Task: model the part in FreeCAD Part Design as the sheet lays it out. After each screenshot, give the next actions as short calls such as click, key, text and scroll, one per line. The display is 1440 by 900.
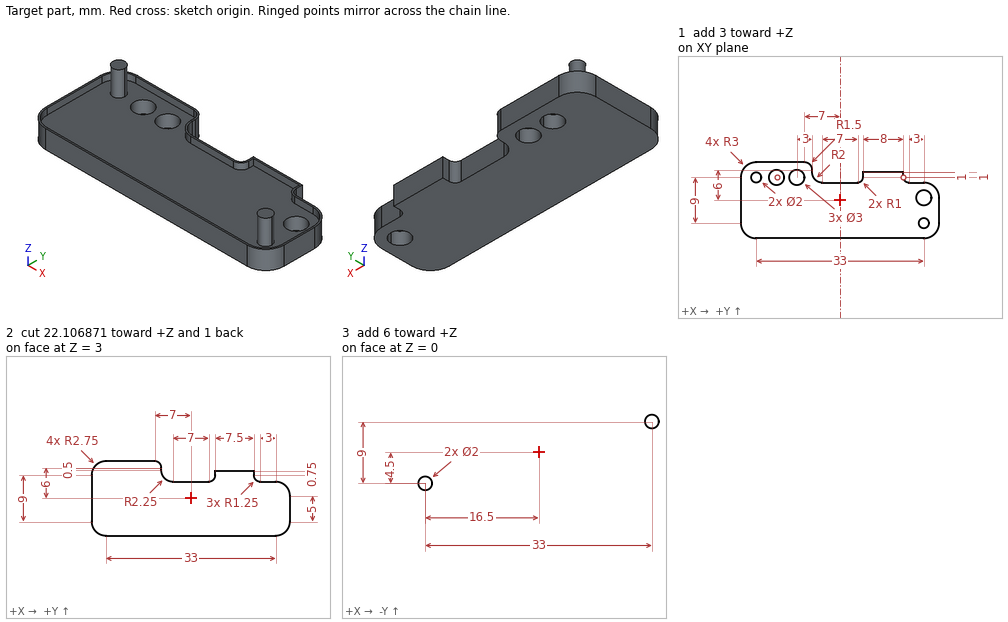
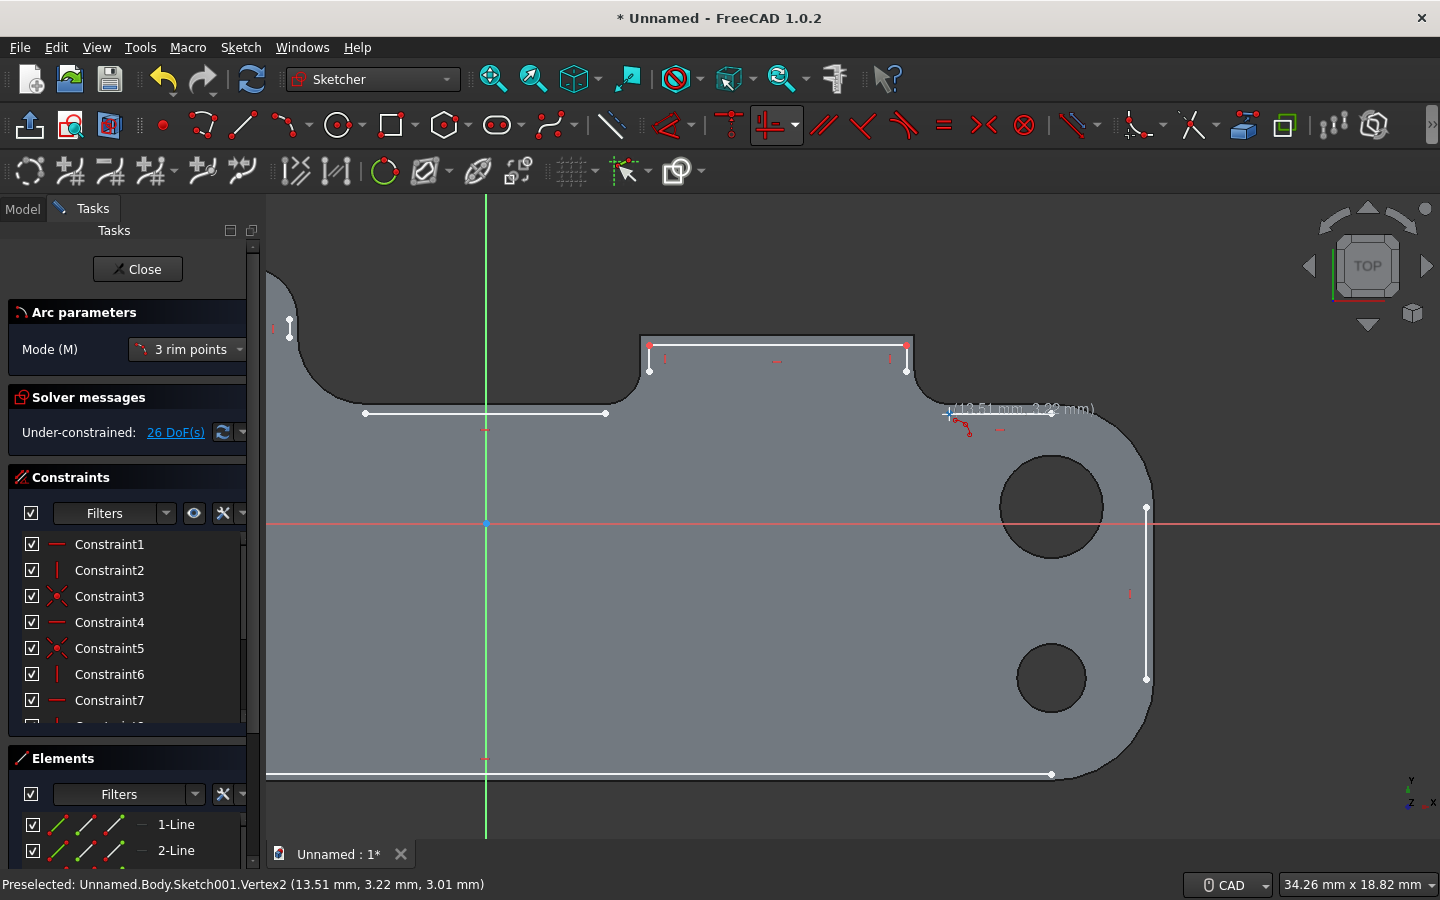
scroll(906, 370, up, 2)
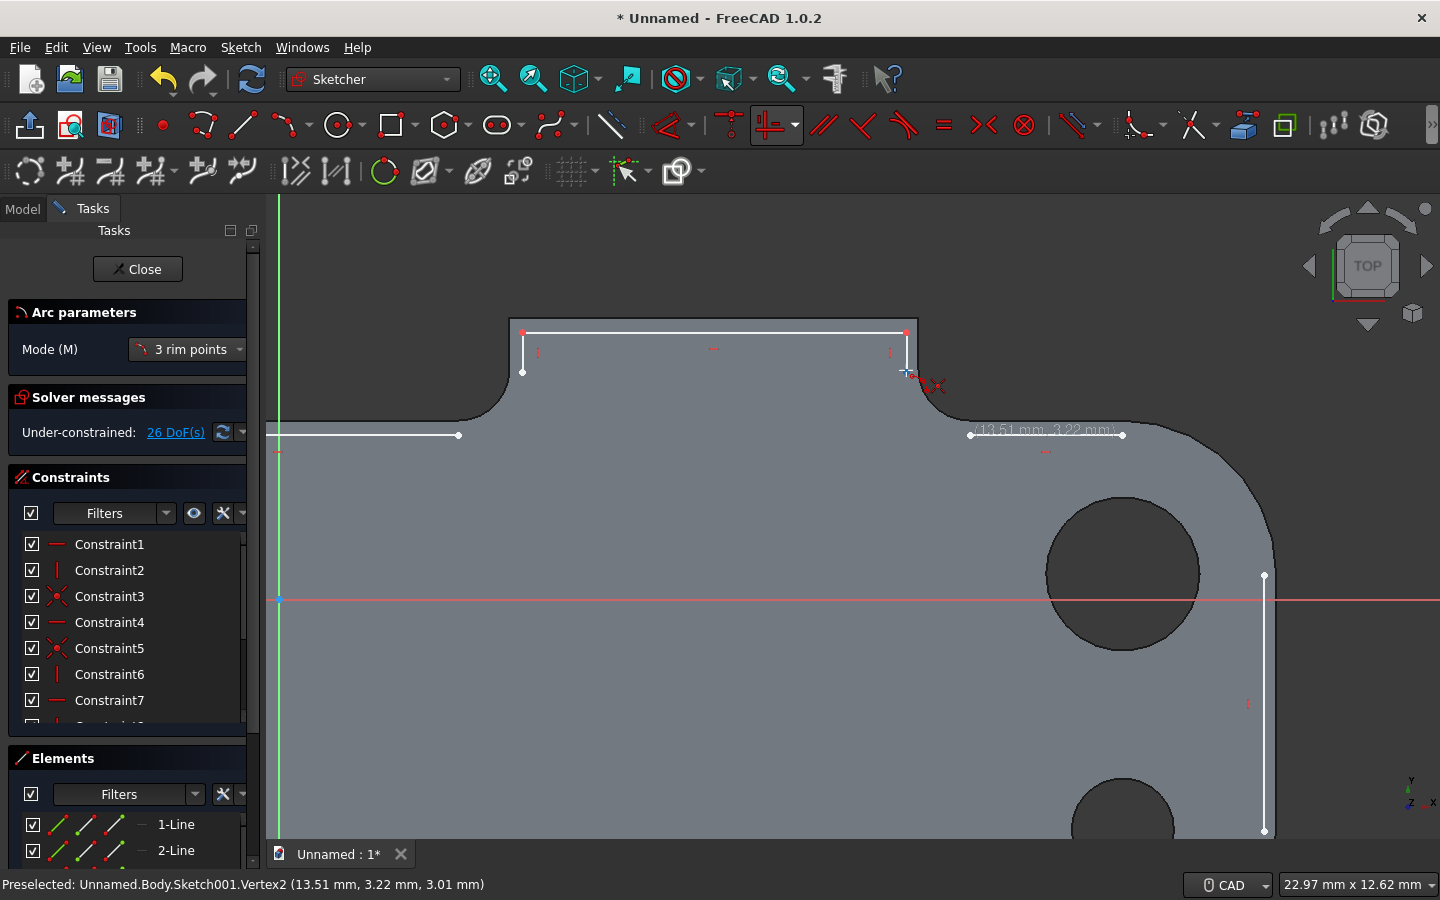
click(907, 372)
click(924, 415)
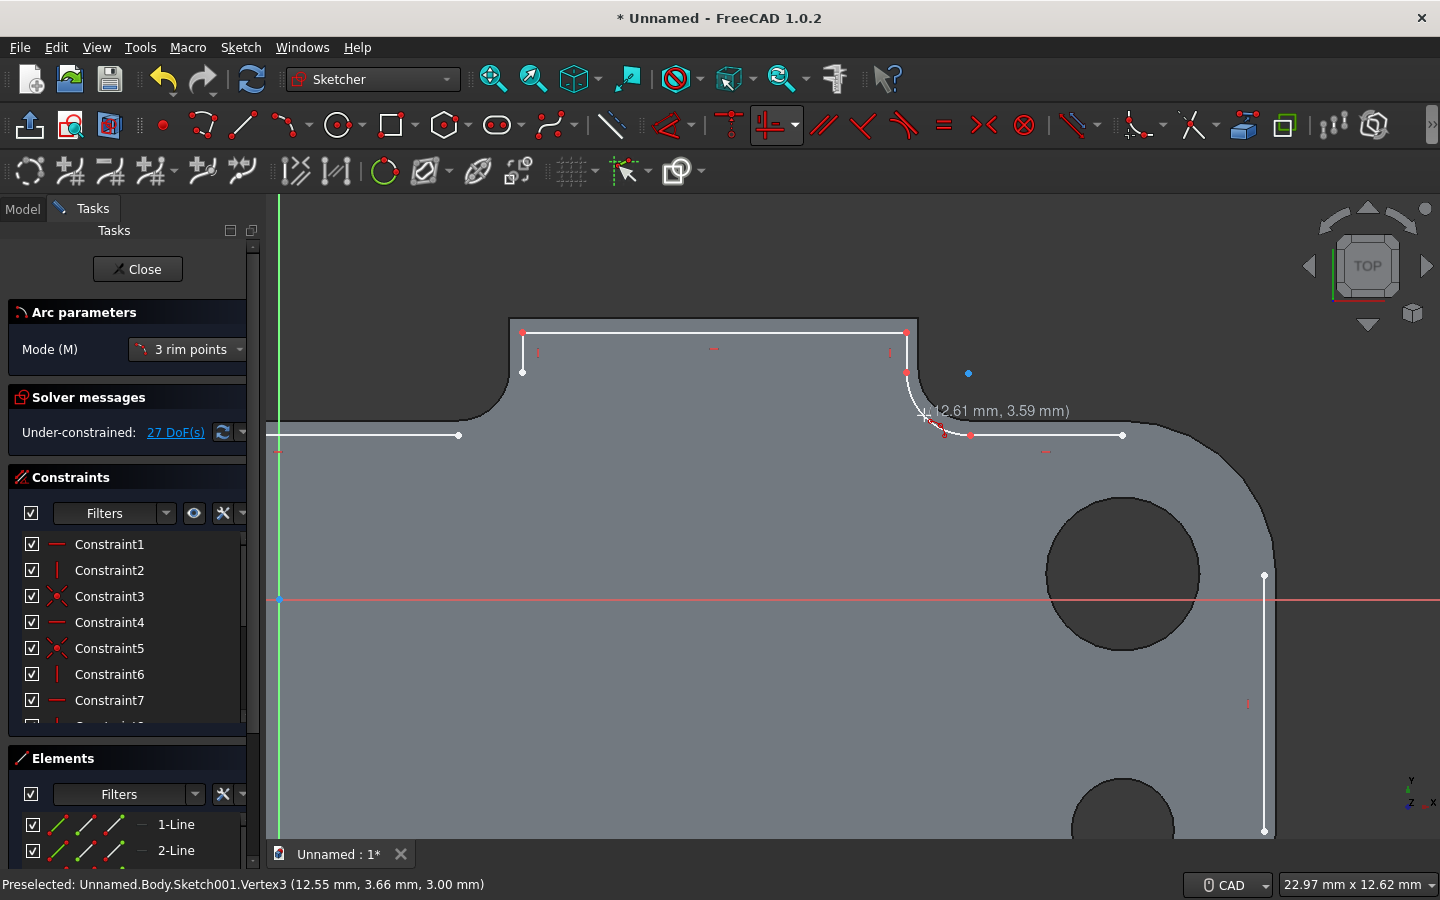
click(523, 373)
click(458, 435)
click(504, 415)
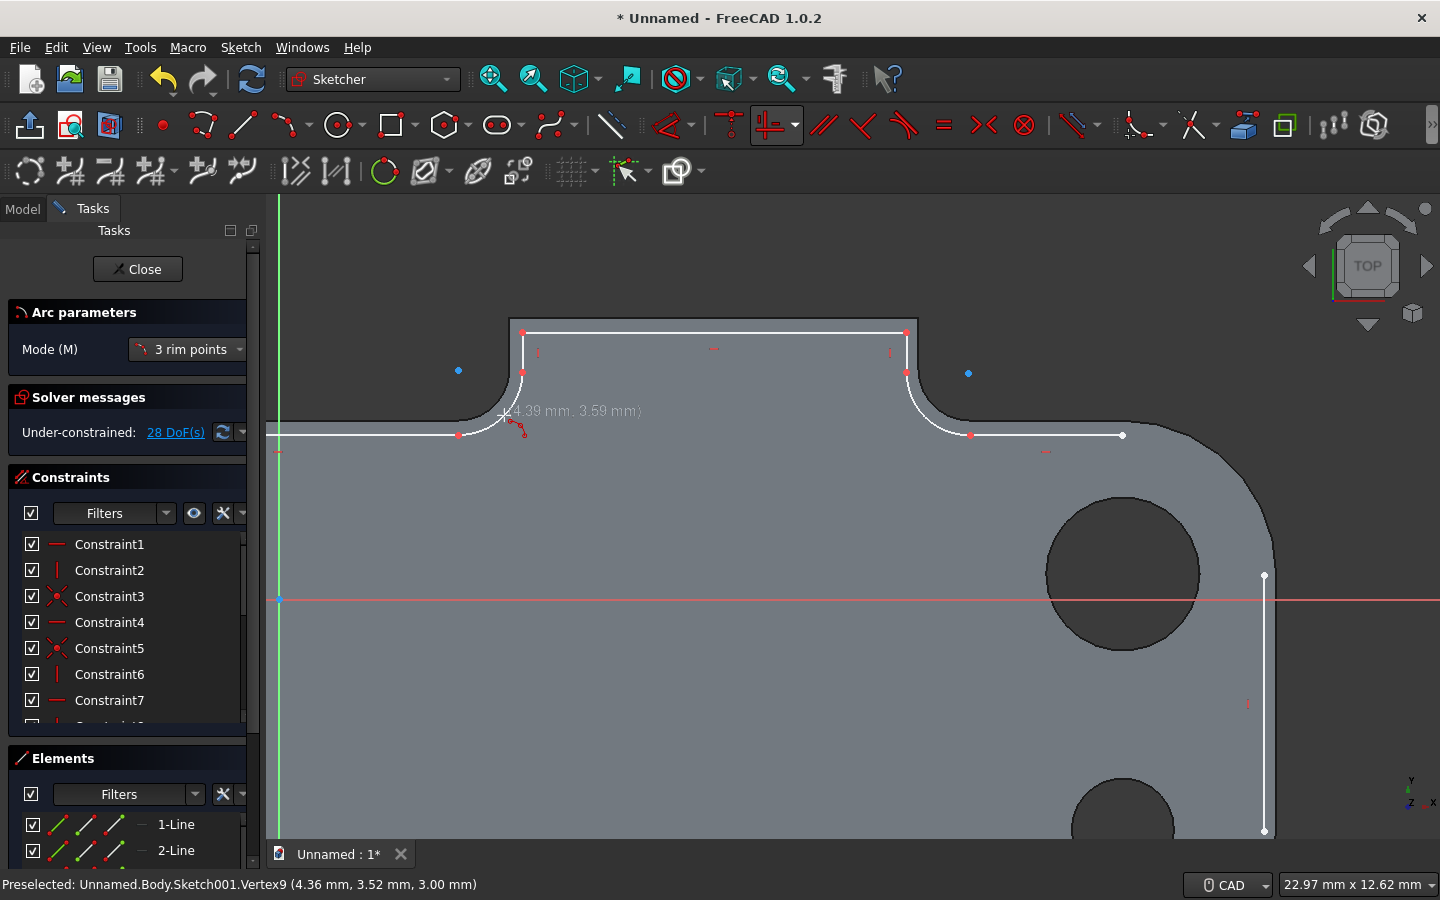
scroll(1078, 468, down, 5)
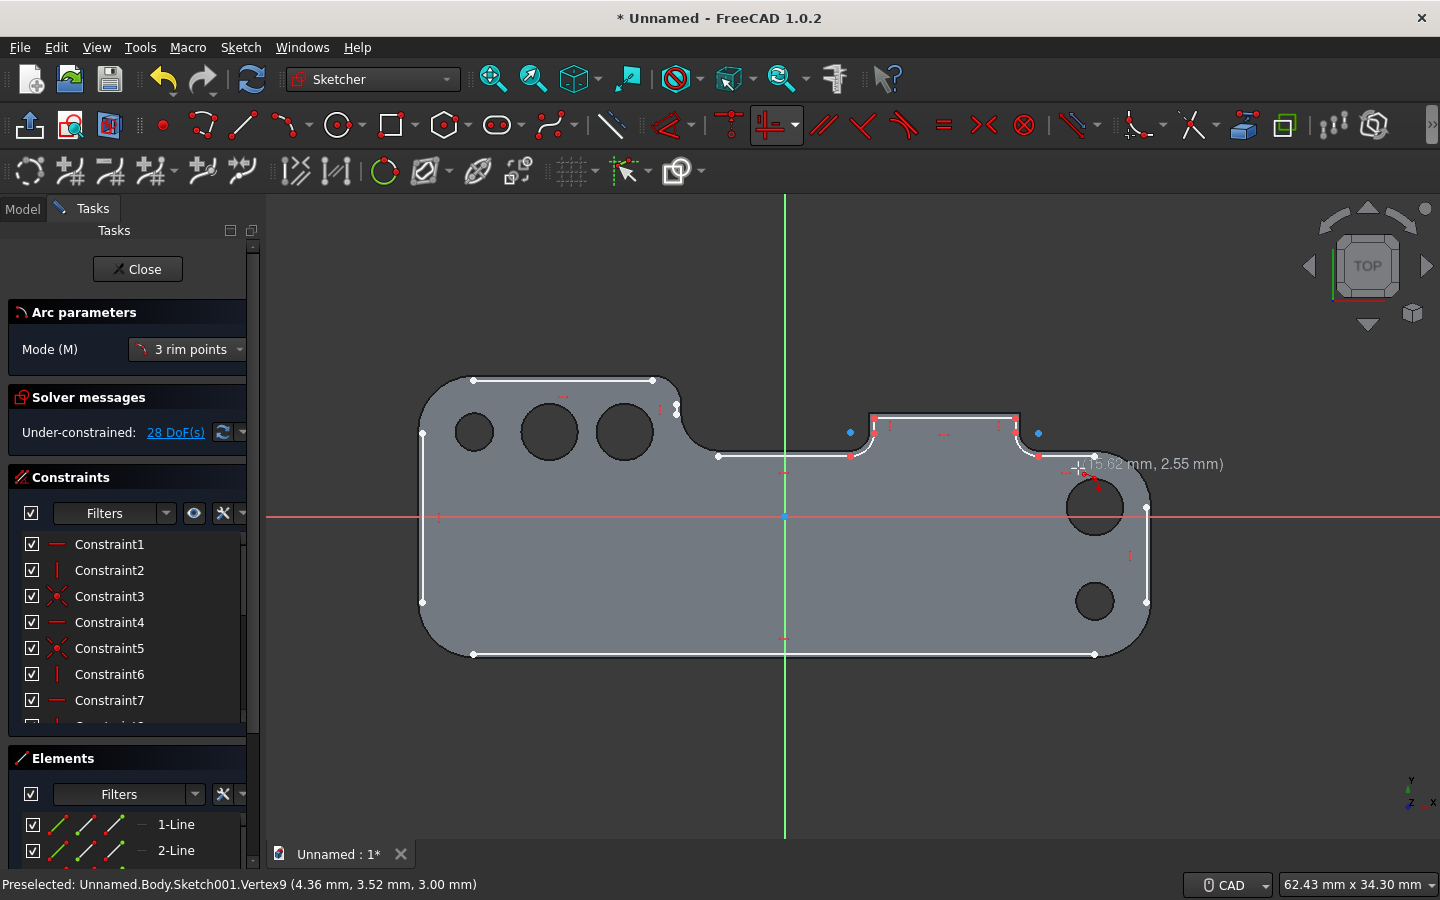
click(719, 456)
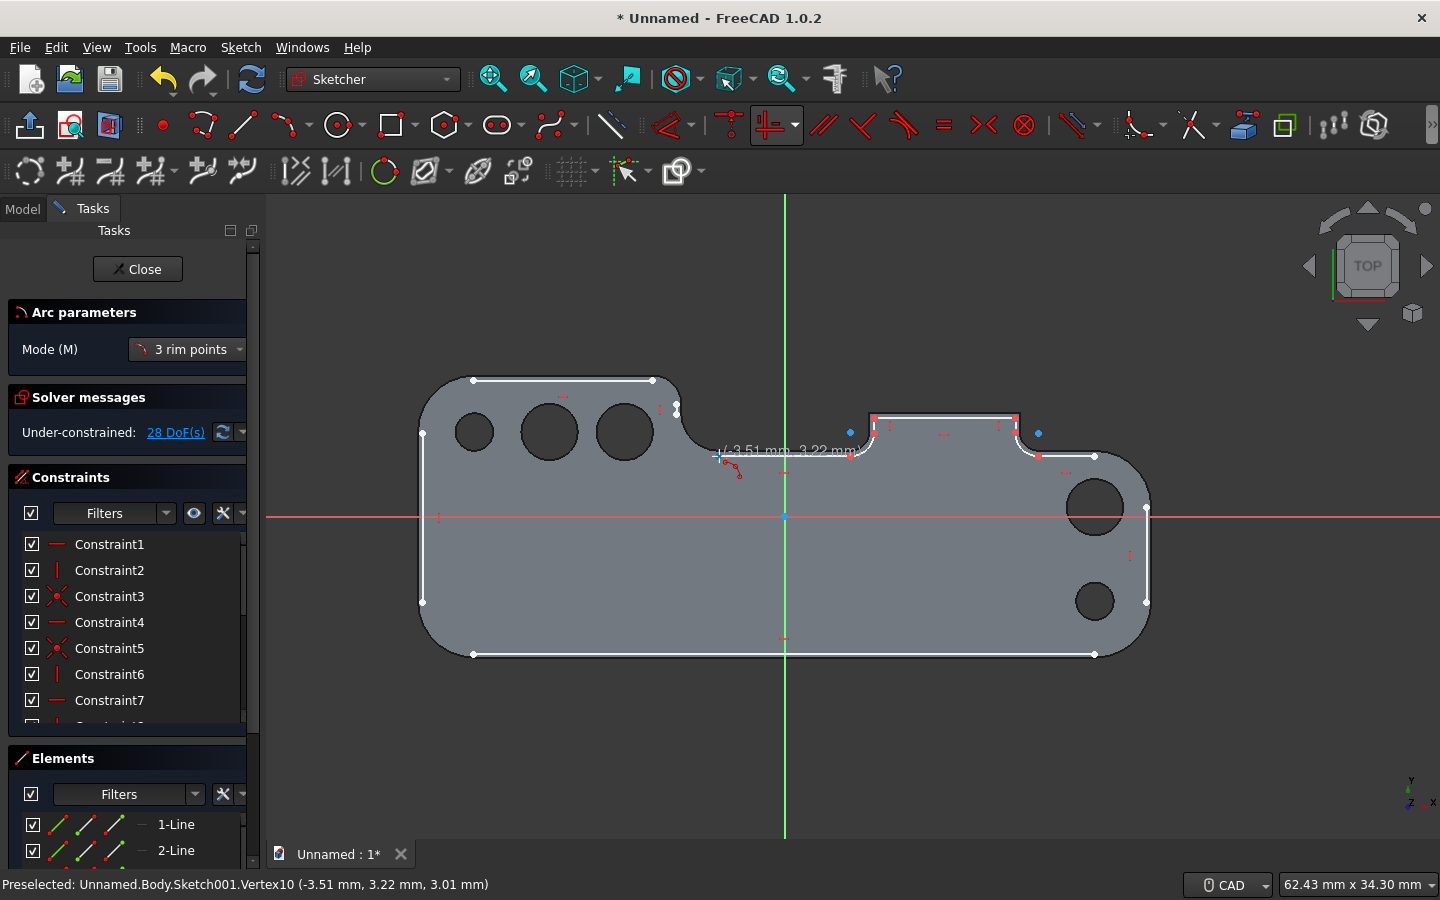
scroll(677, 413, up, 7)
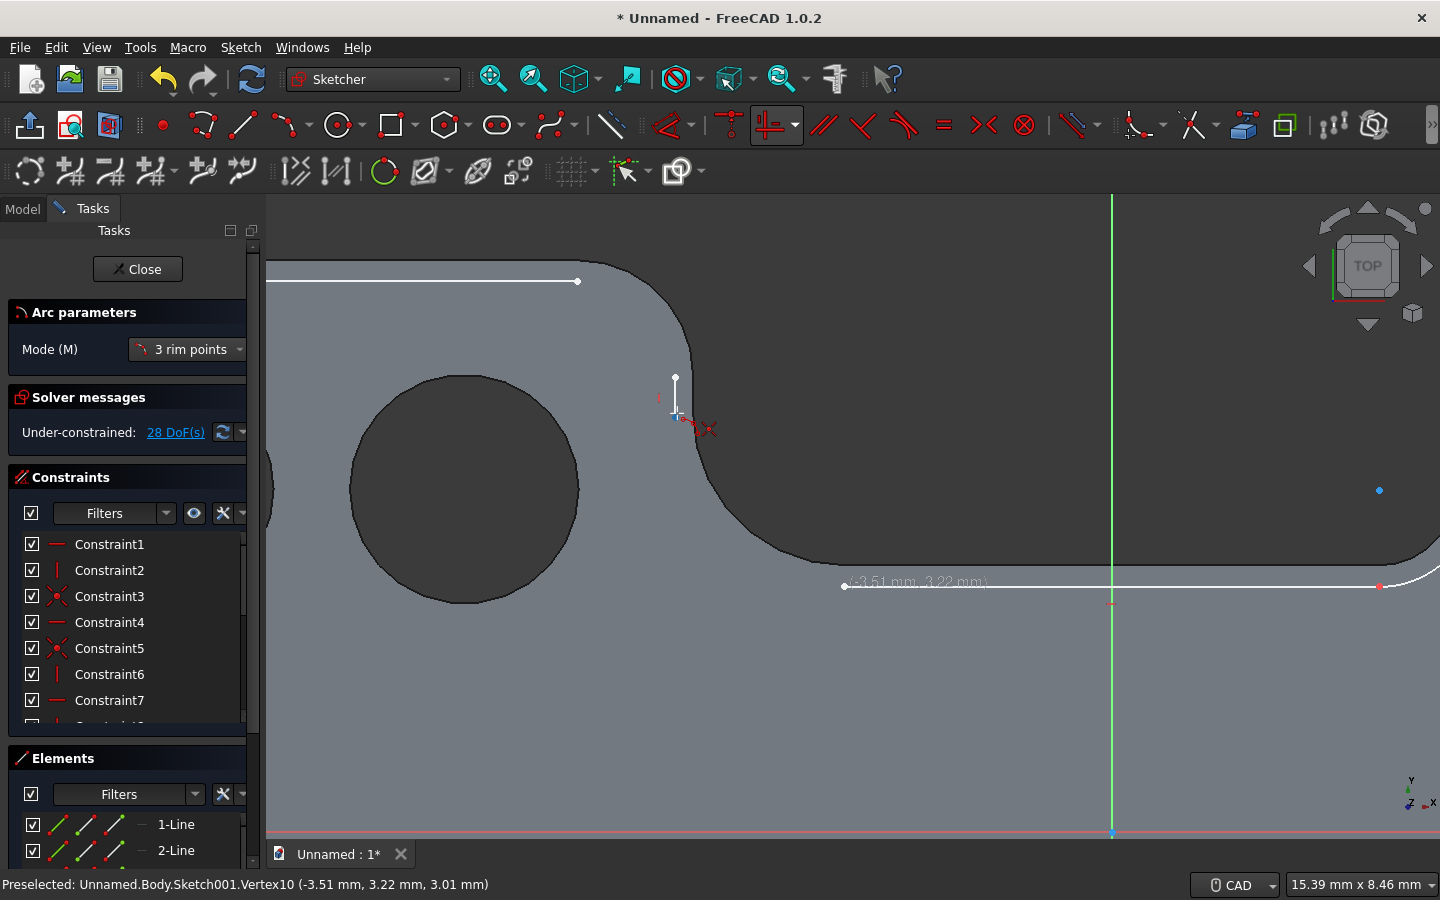
click(675, 418)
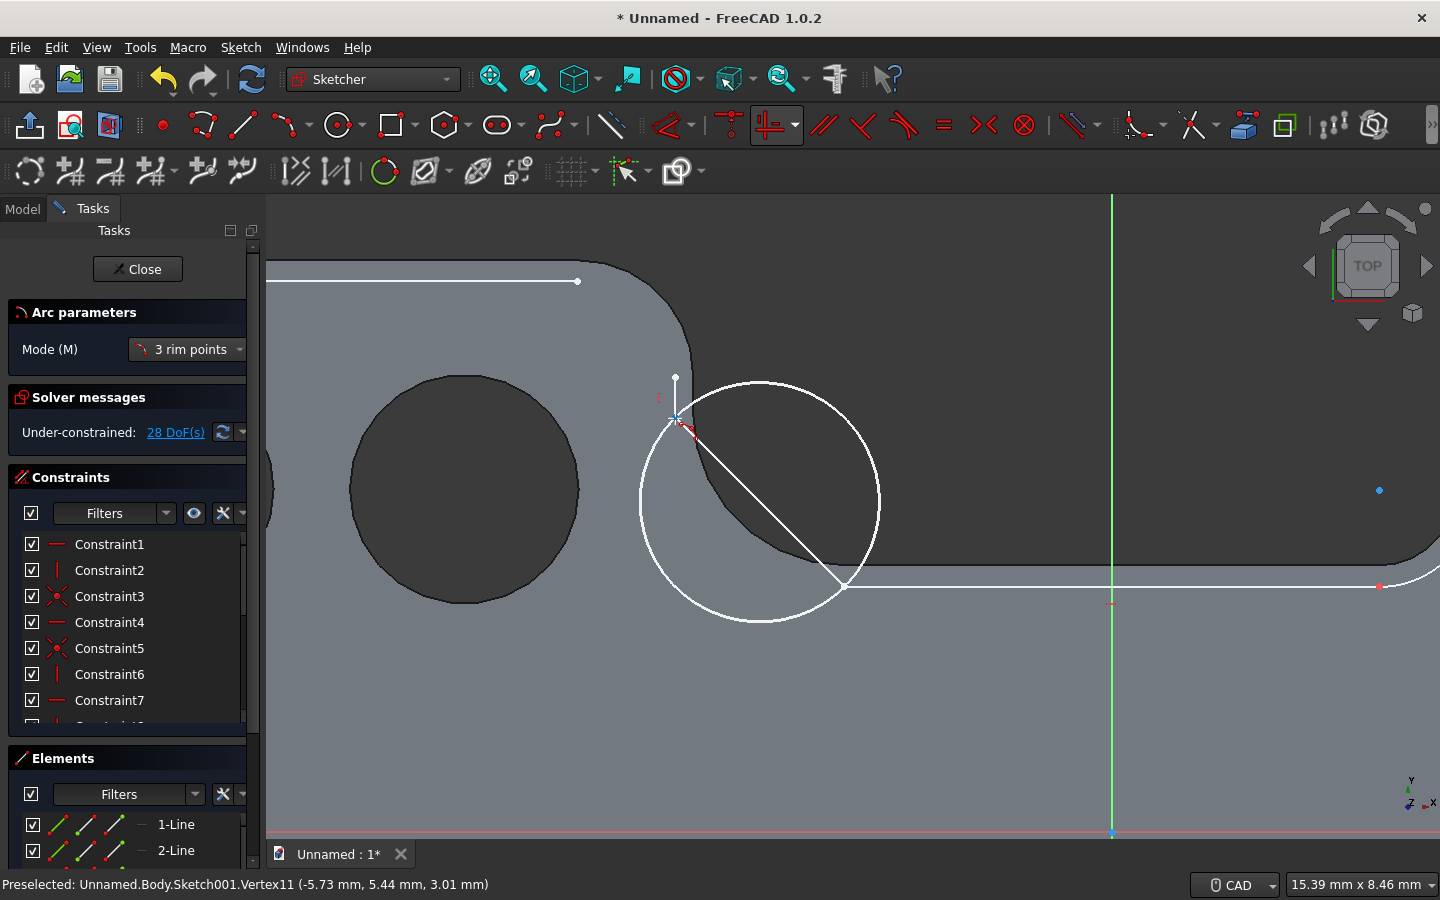
scroll(677, 413, down, 7)